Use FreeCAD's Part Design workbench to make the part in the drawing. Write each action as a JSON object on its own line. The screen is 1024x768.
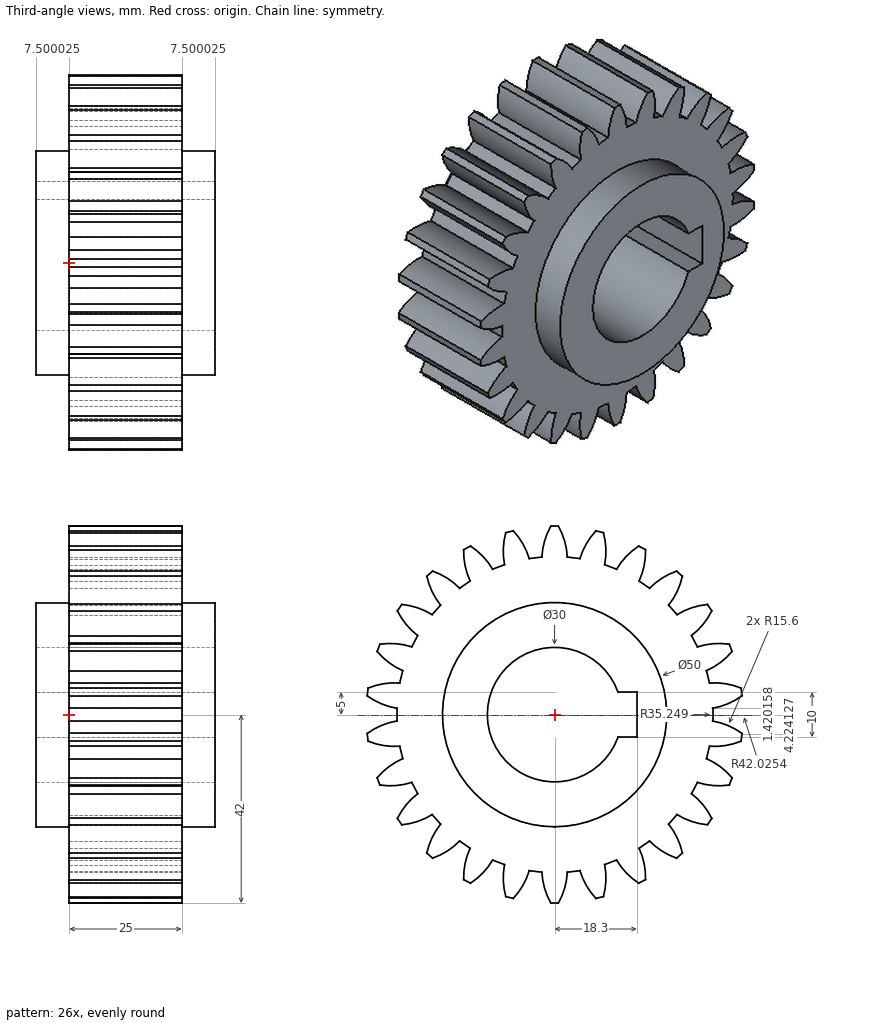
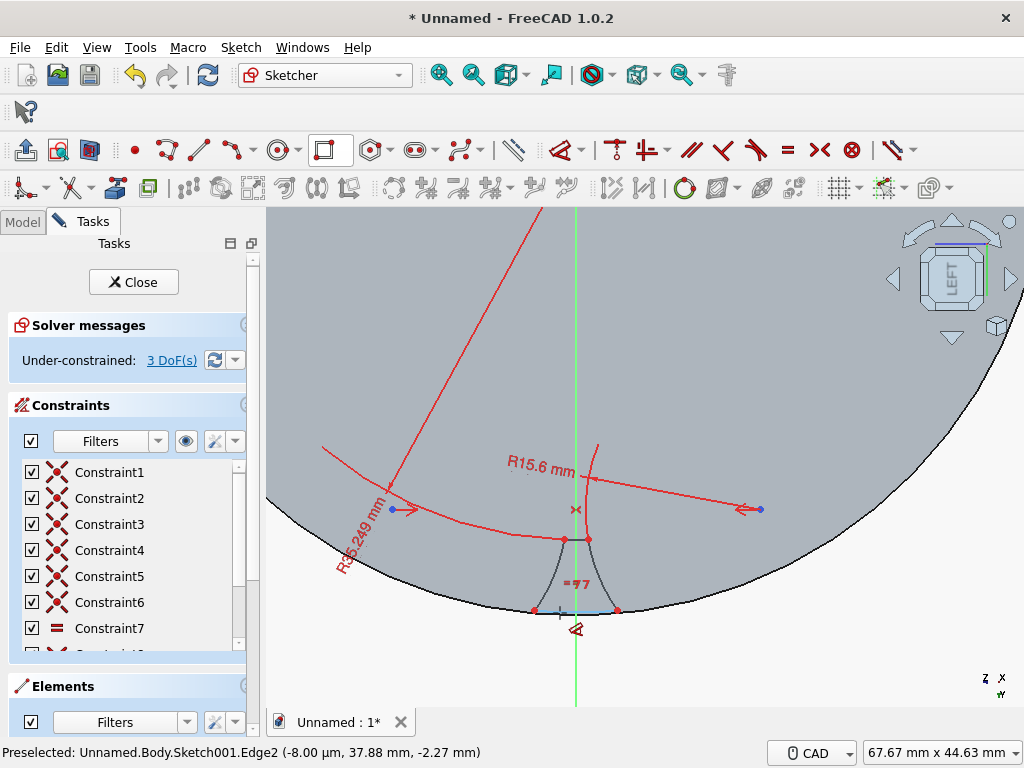
{"action": "left_click", "coordinate": [560, 612]}
{"action": "left_click", "coordinate": [559, 644]}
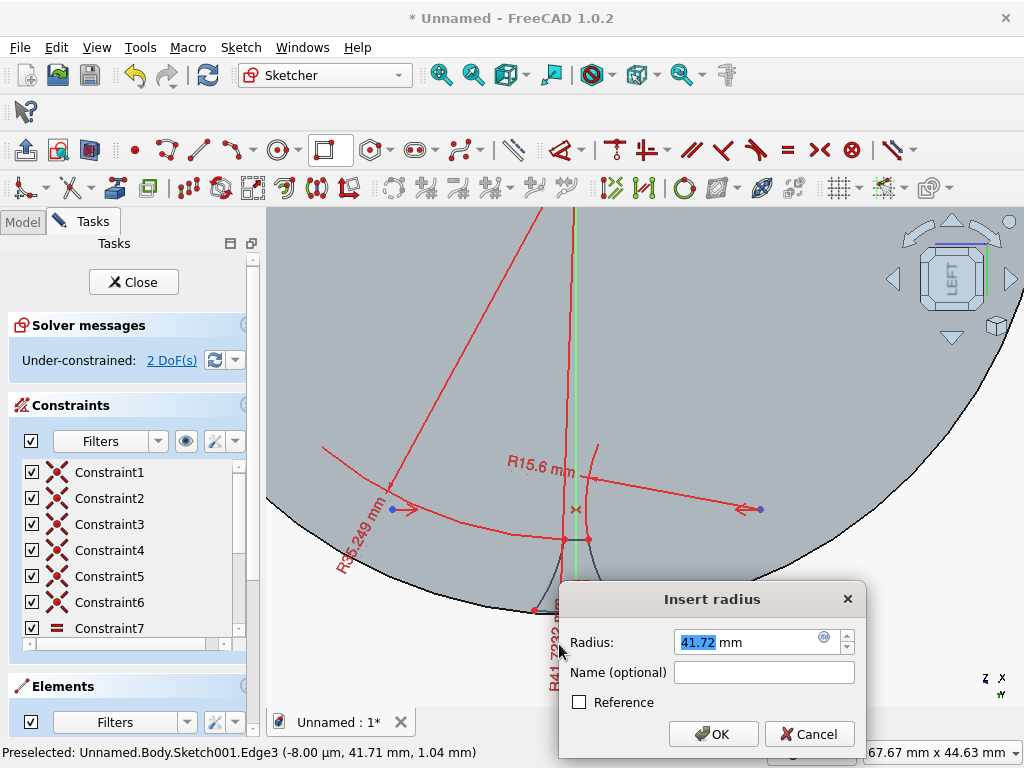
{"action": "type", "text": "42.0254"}
{"action": "key", "text": "Return"}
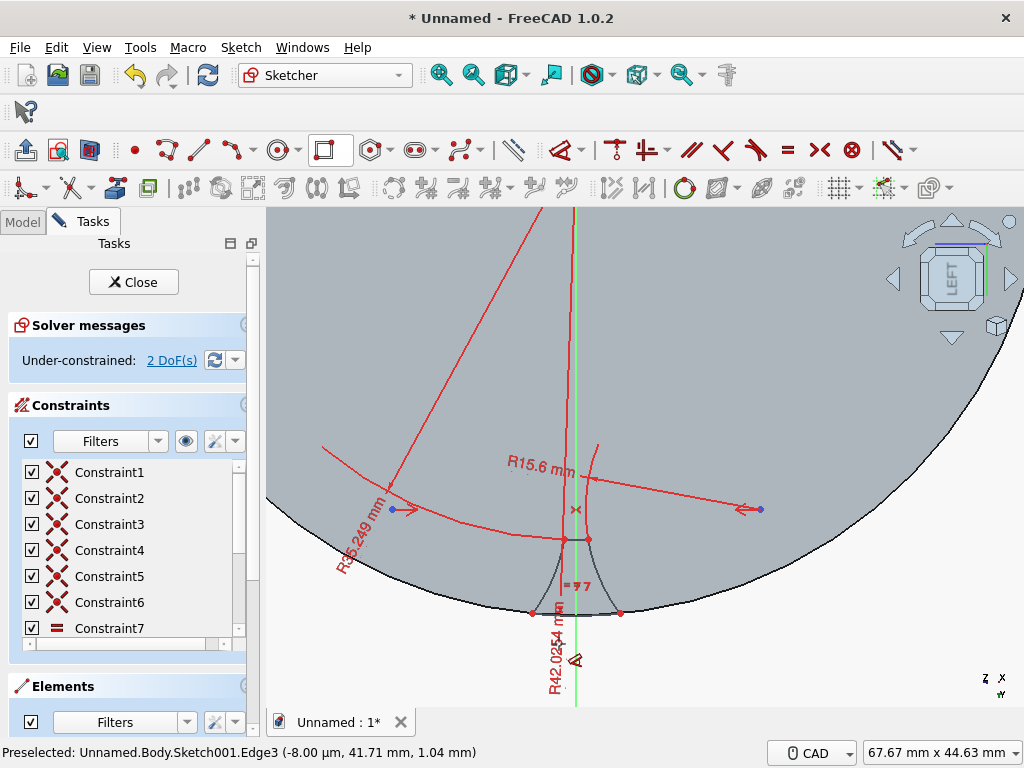
{"action": "scroll", "coordinate": [564, 540], "scroll_direction": "up", "scroll_amount": 5}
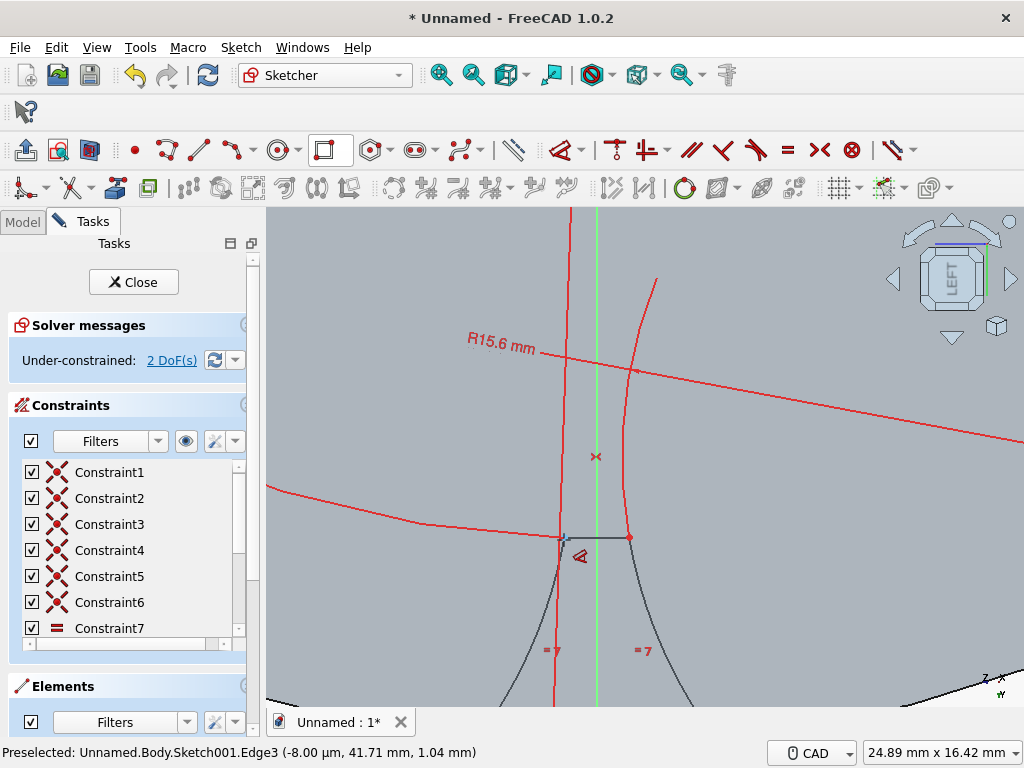
{"action": "left_click", "coordinate": [564, 538]}
{"action": "left_click", "coordinate": [580, 572]}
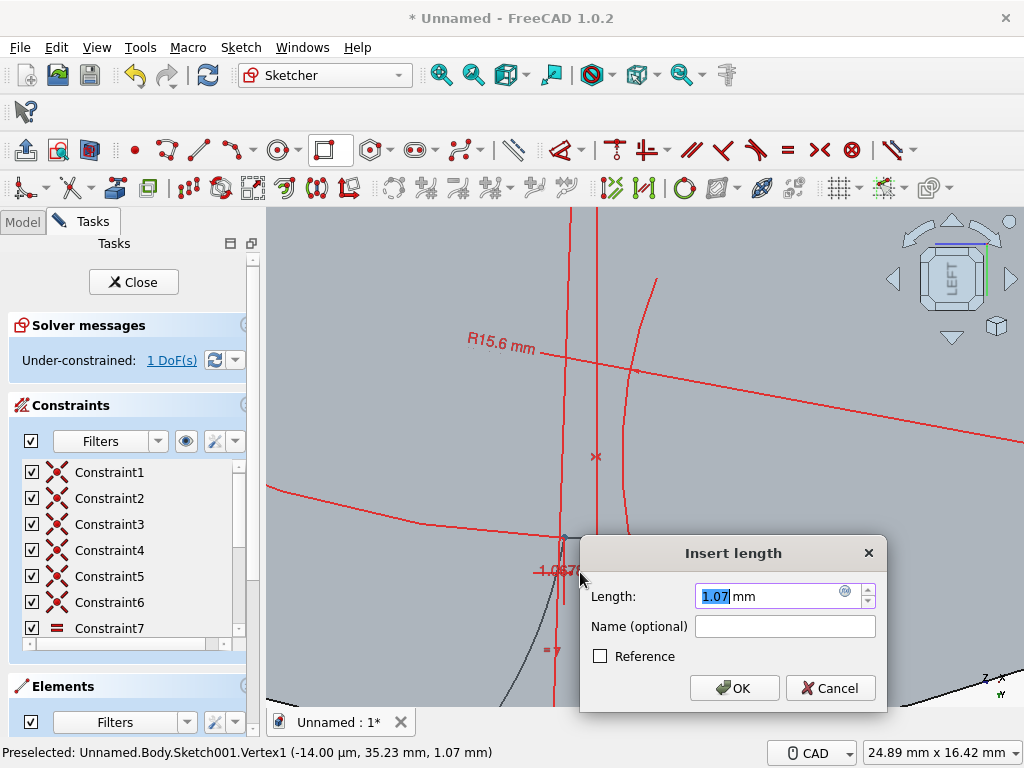
{"action": "type", "text": "1.420158"}
{"action": "key", "text": "Return"}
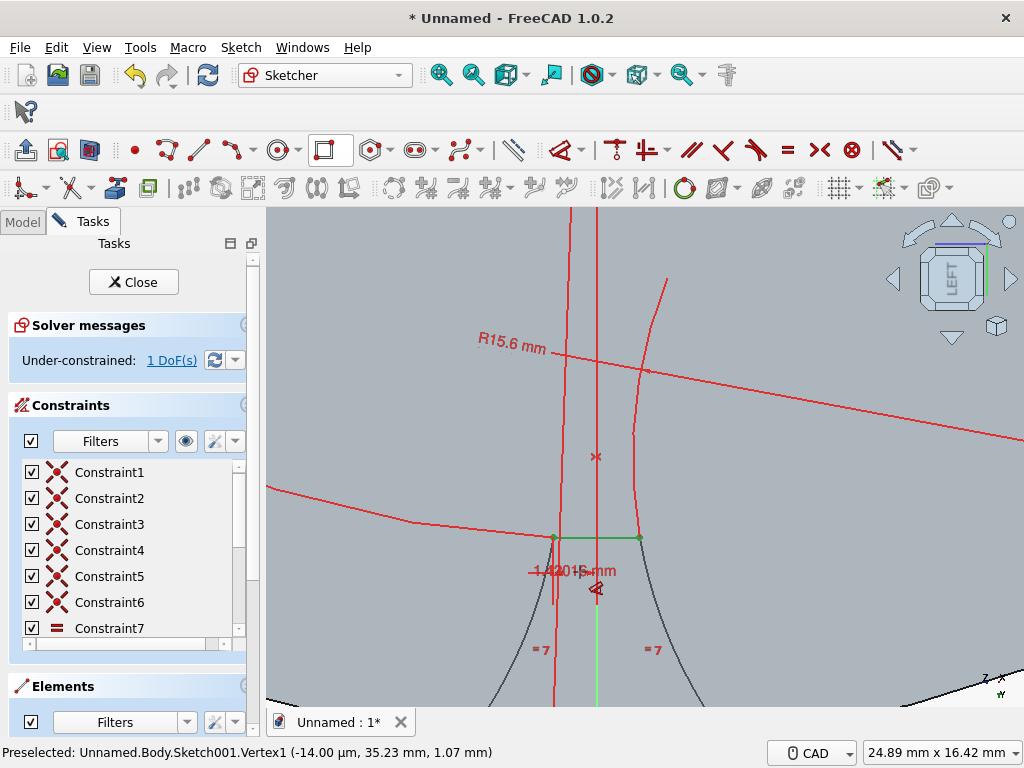
{"action": "scroll", "coordinate": [485, 235], "scroll_direction": "down", "scroll_amount": 1}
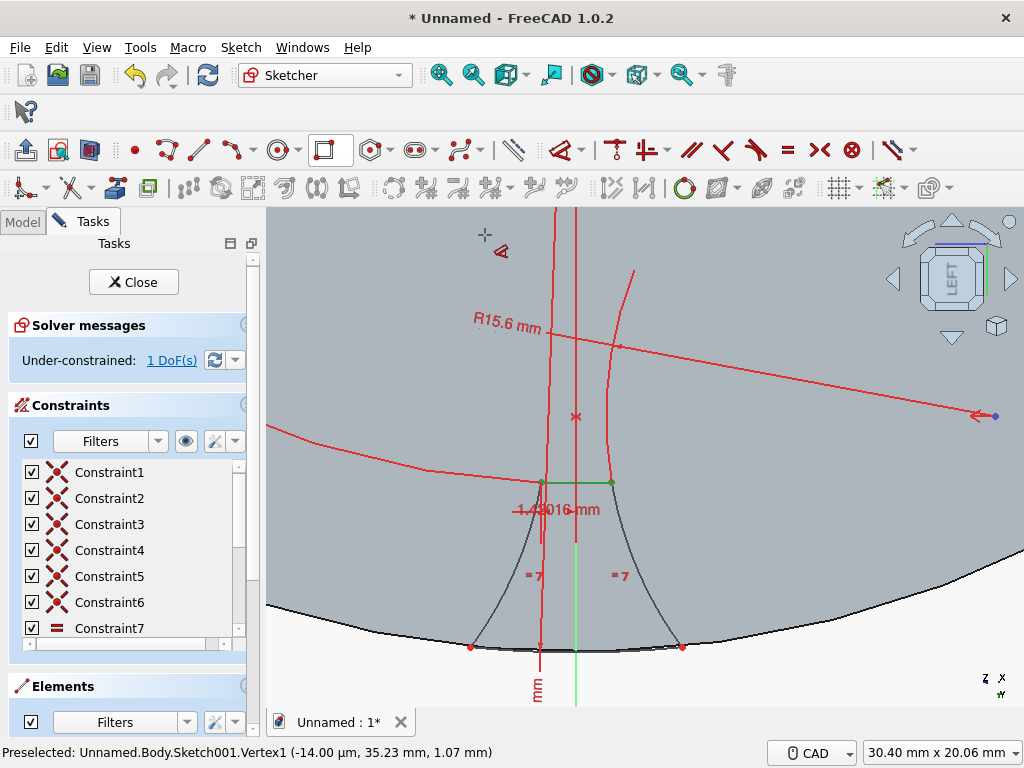
{"action": "scroll", "coordinate": [576, 679], "scroll_direction": "up", "scroll_amount": 3}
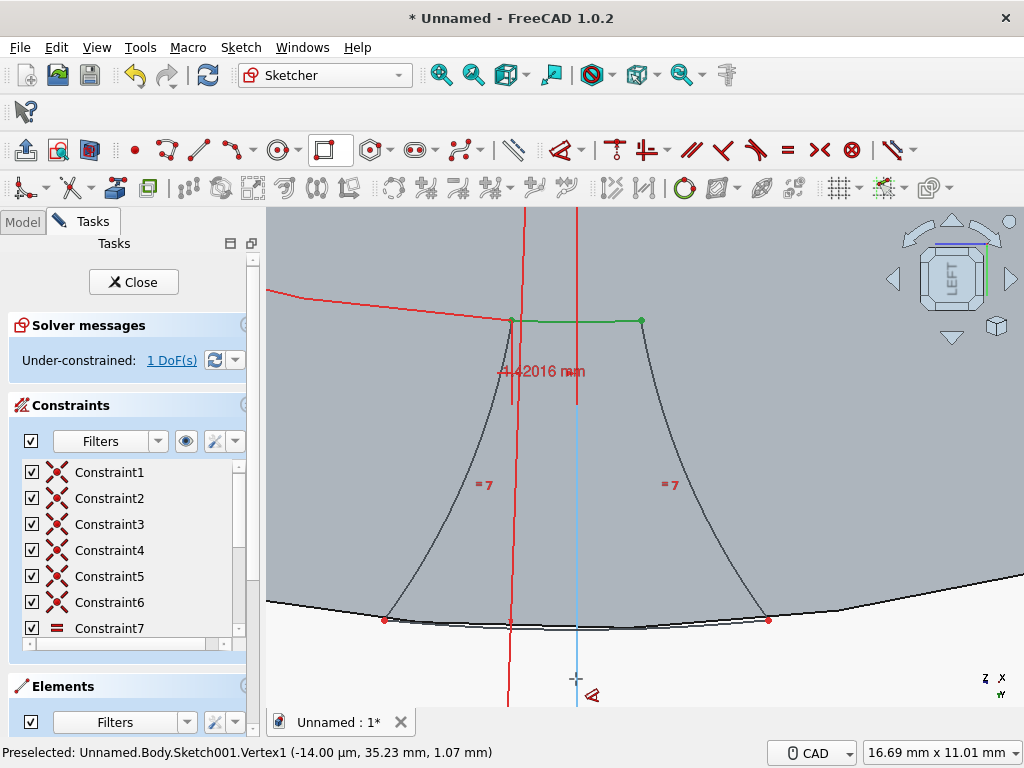
{"action": "left_click", "coordinate": [769, 620]}
{"action": "left_click", "coordinate": [673, 654]}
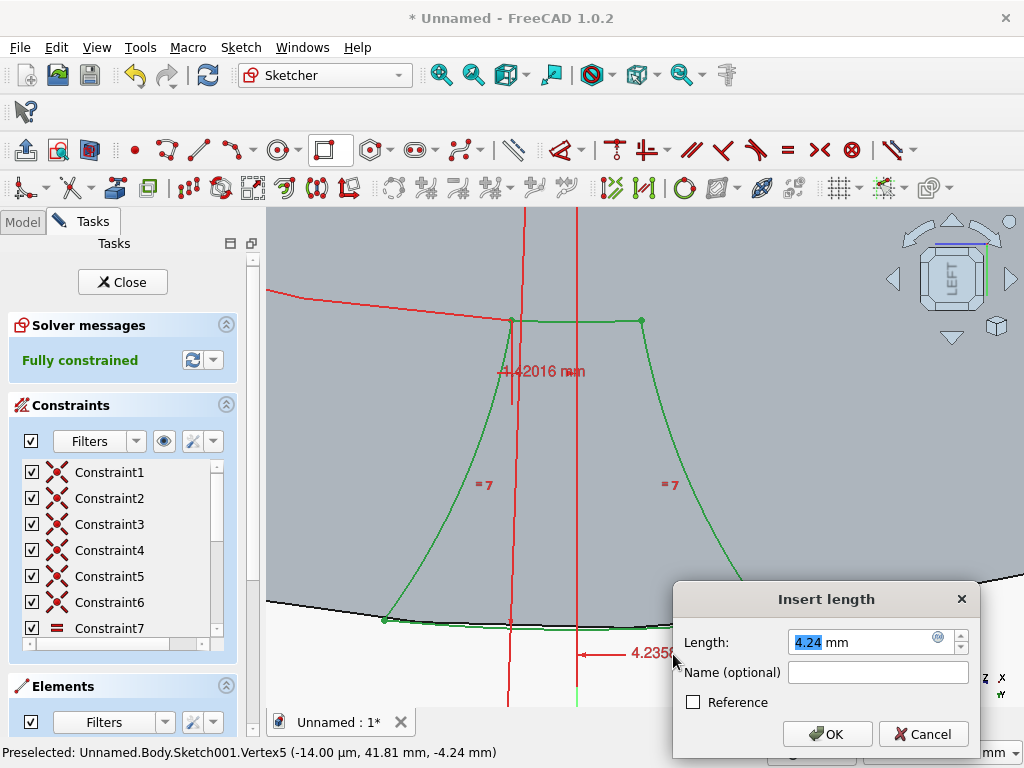
{"action": "type", "text": "4.224127"}
{"action": "key", "text": "Return"}
{"action": "key", "text": "Escape"}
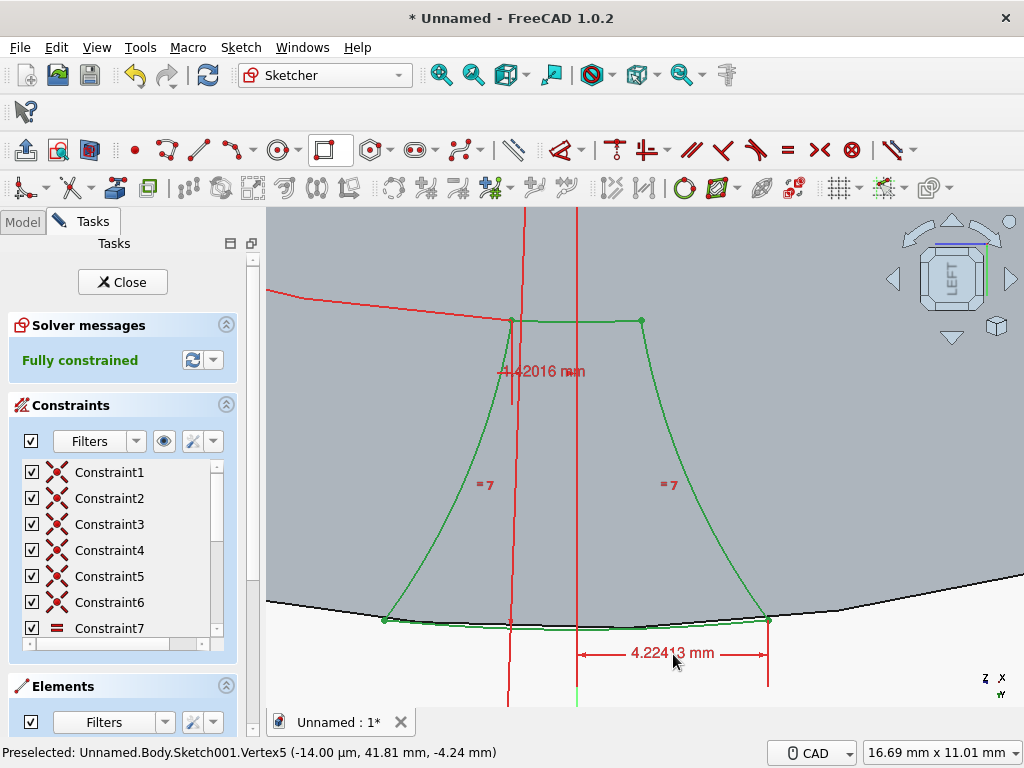
{"action": "left_click", "coordinate": [123, 282]}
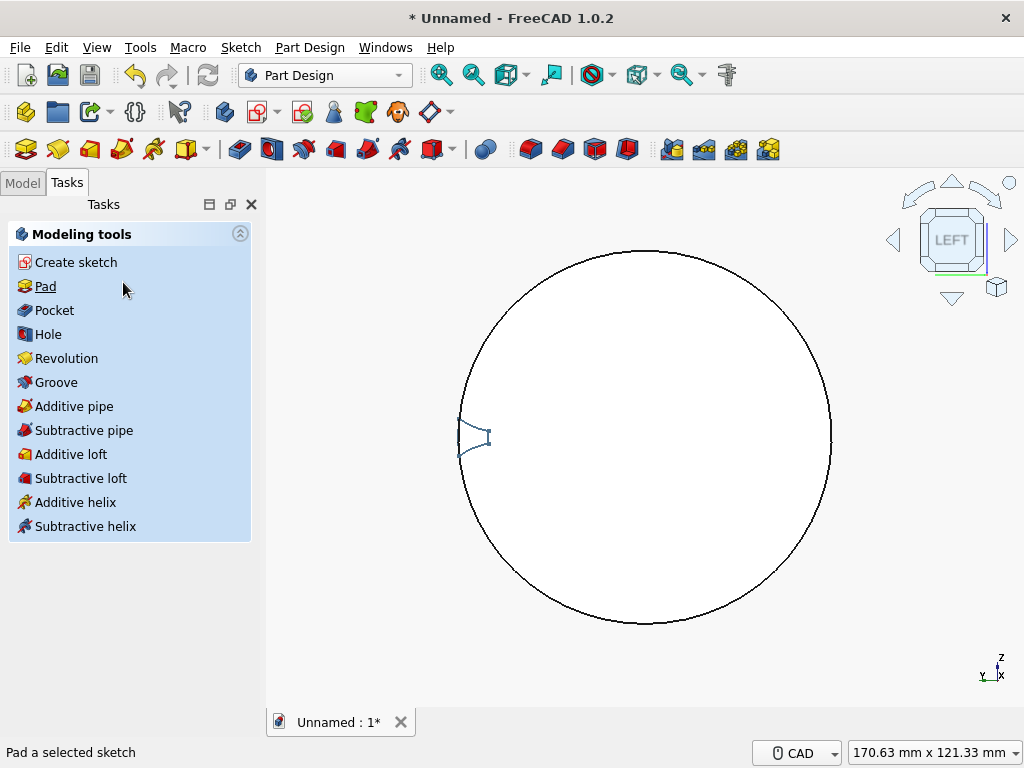
{"action": "left_click", "coordinate": [240, 150]}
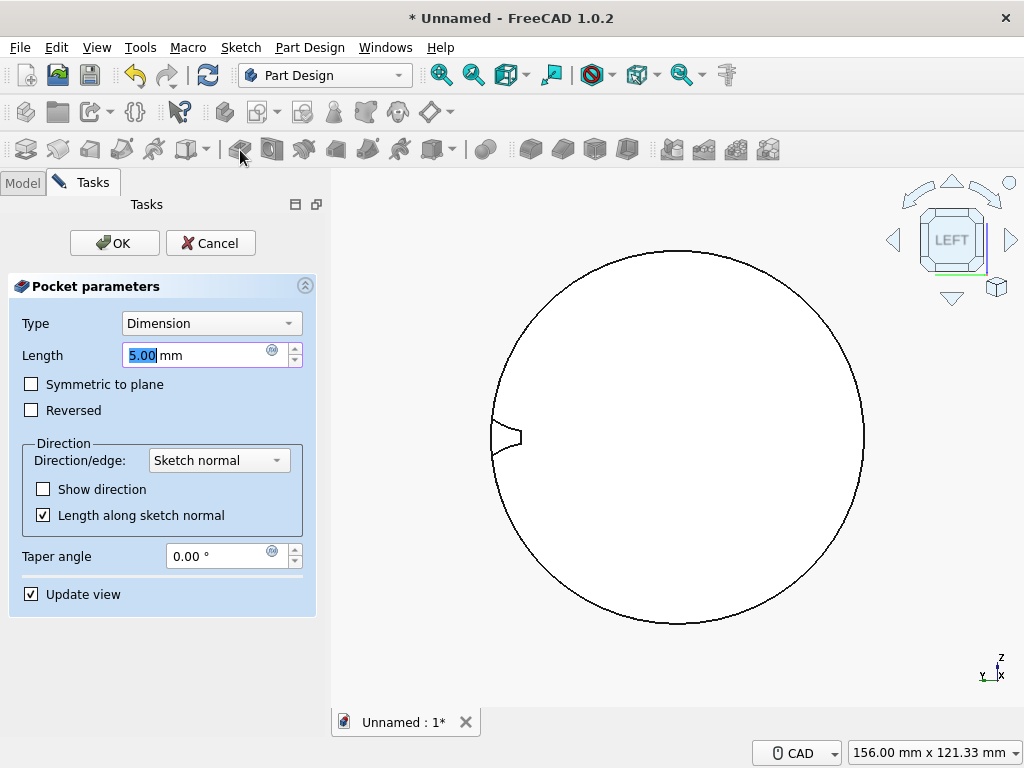
{"action": "left_click", "coordinate": [212, 324]}